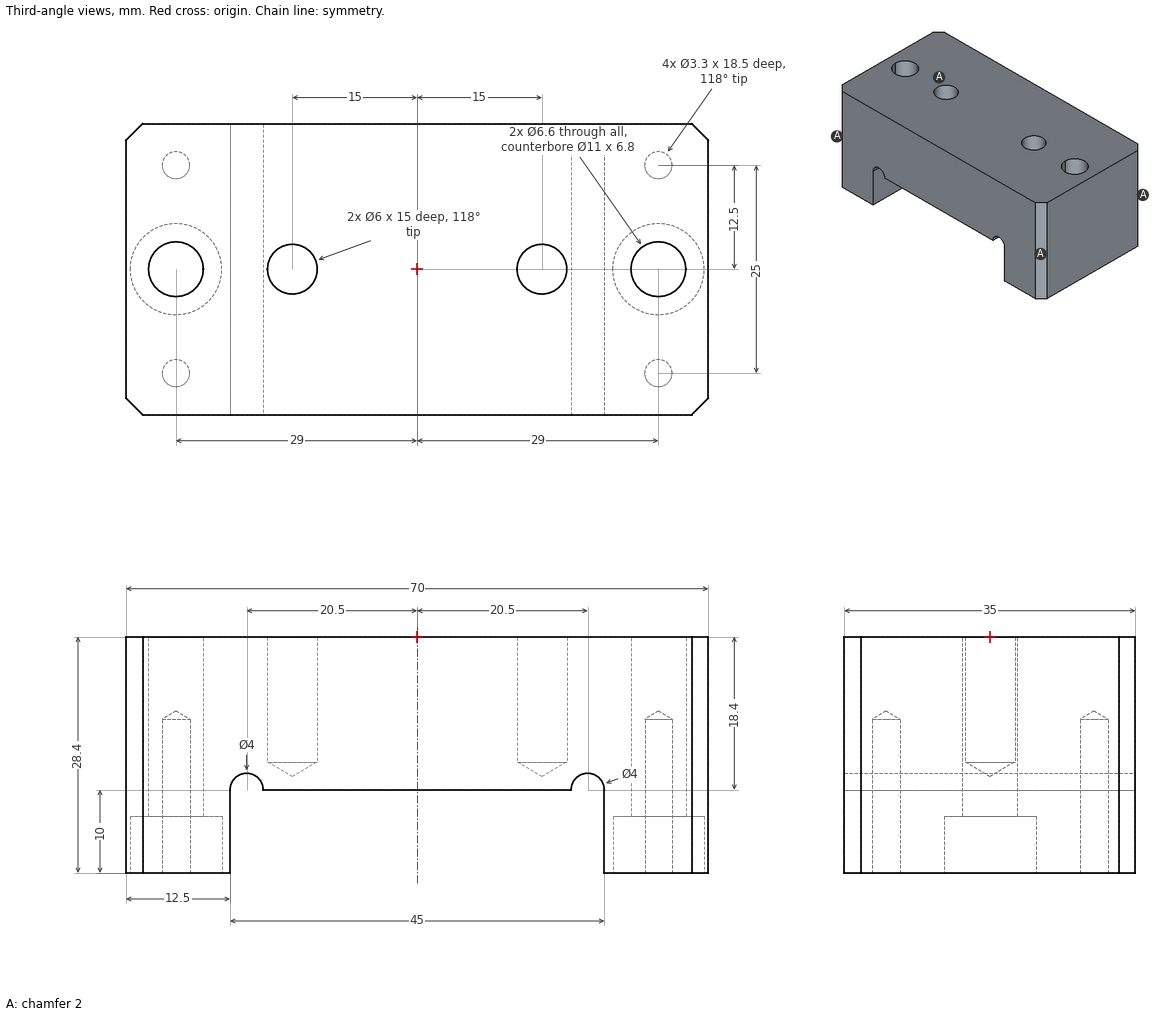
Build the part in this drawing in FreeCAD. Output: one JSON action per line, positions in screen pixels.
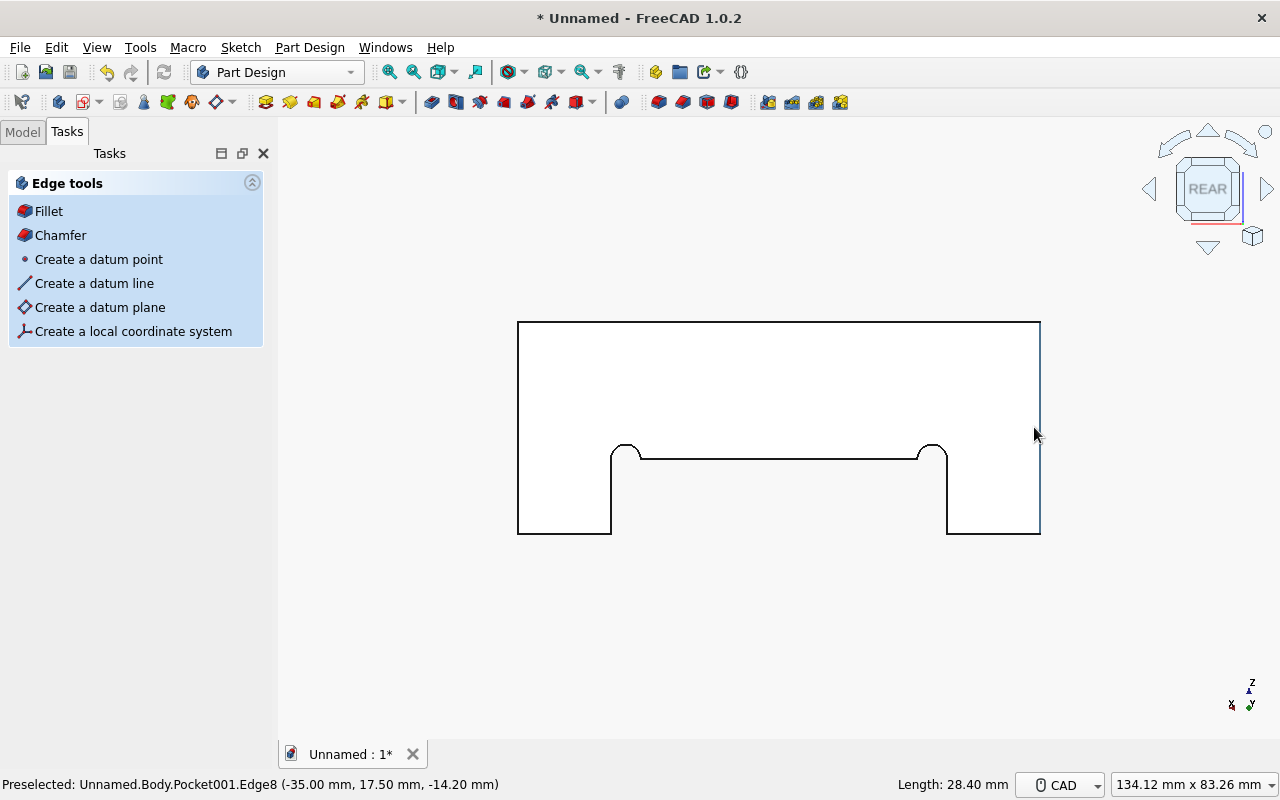
{"action": "key", "text": "0"}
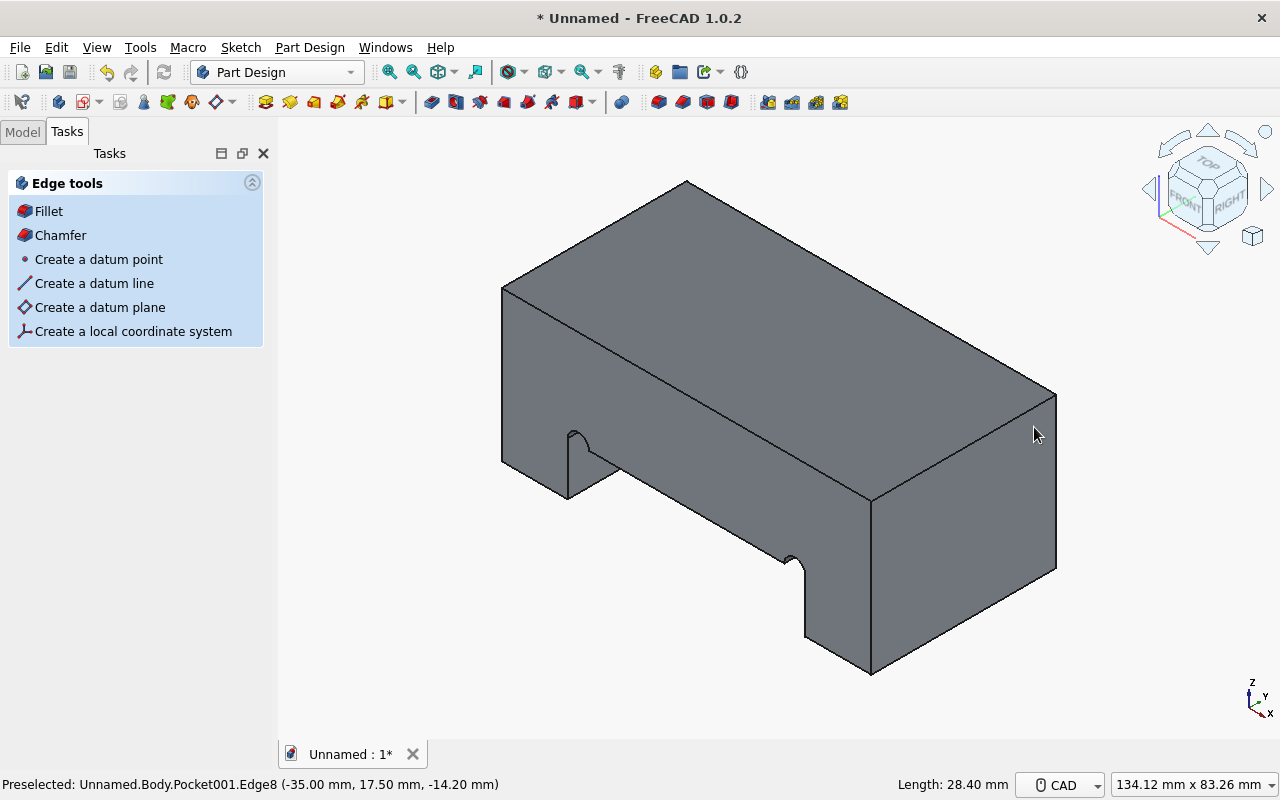
{"action": "left_click", "coordinate": [871, 587], "text": "ctrl"}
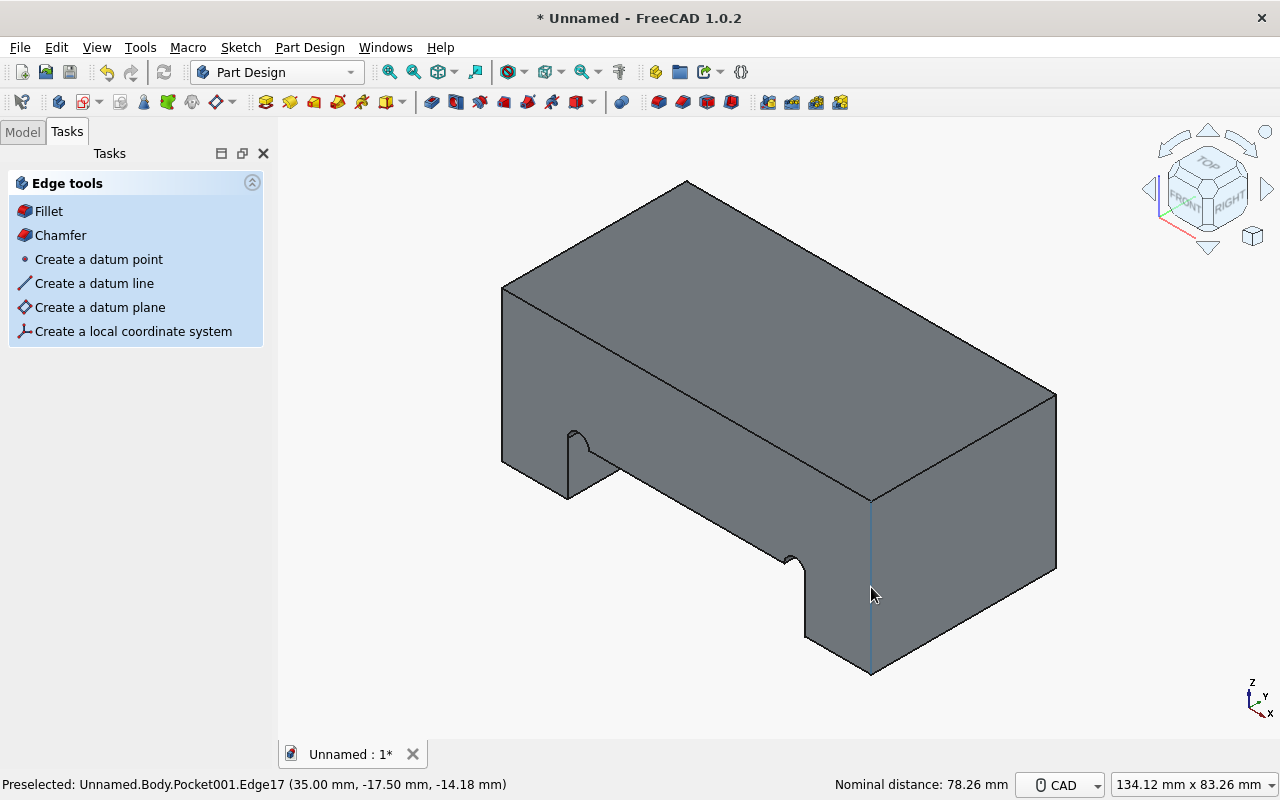
{"action": "key", "text": "2"}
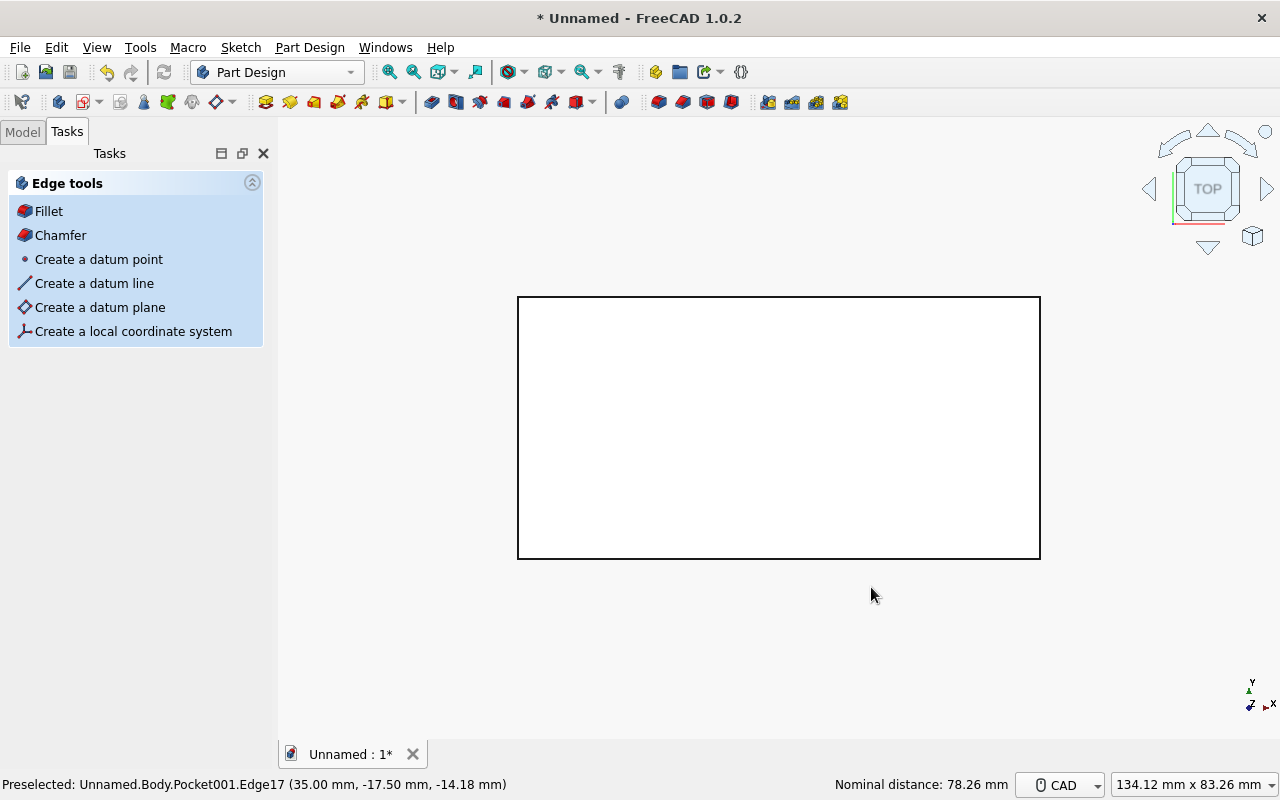
{"action": "key", "text": "1"}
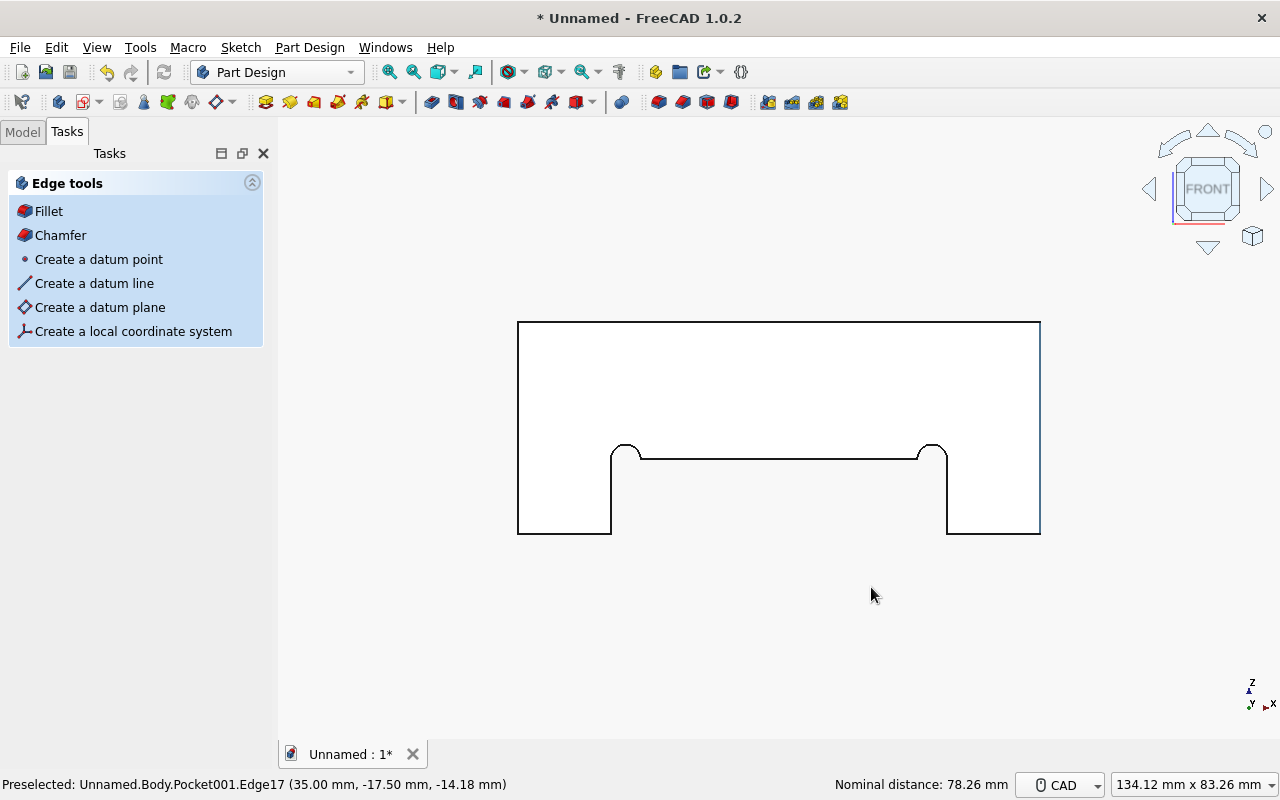
{"action": "left_click", "coordinate": [518, 427], "text": "ctrl"}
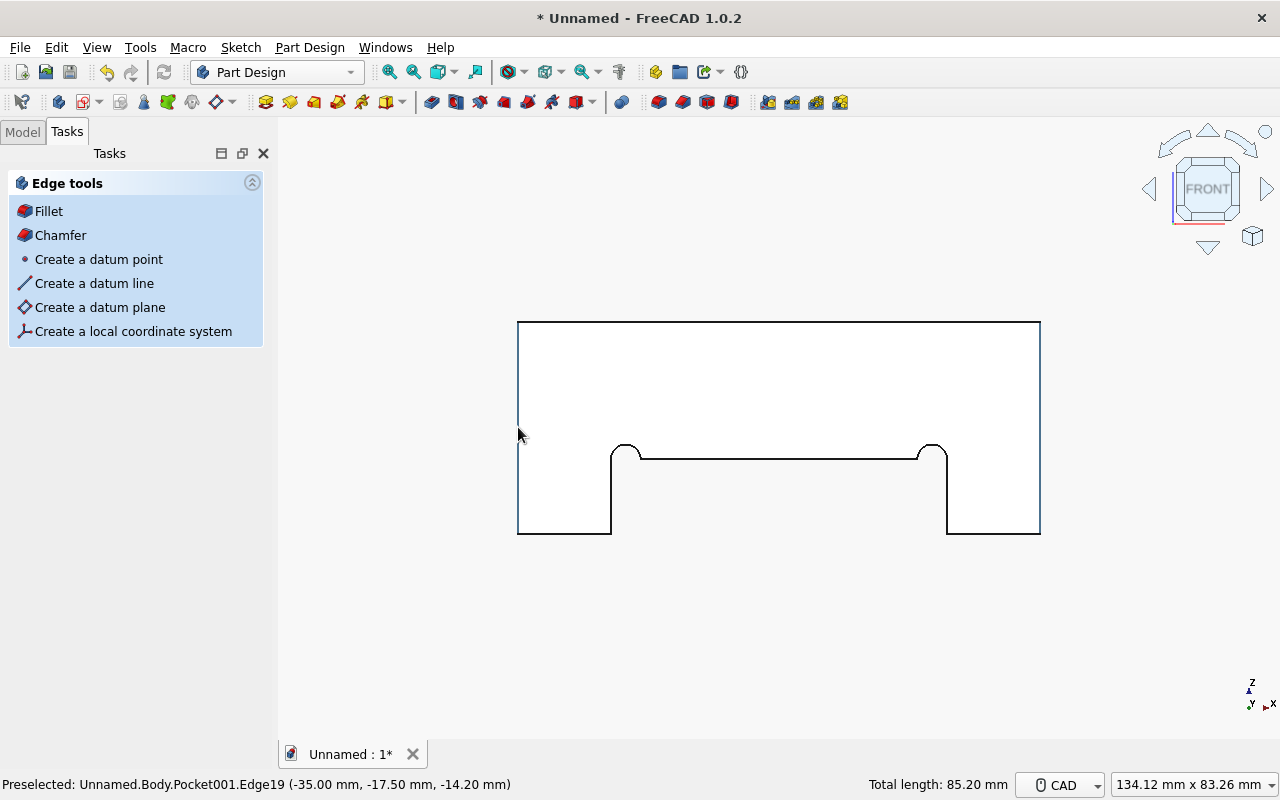
{"action": "key", "text": "3"}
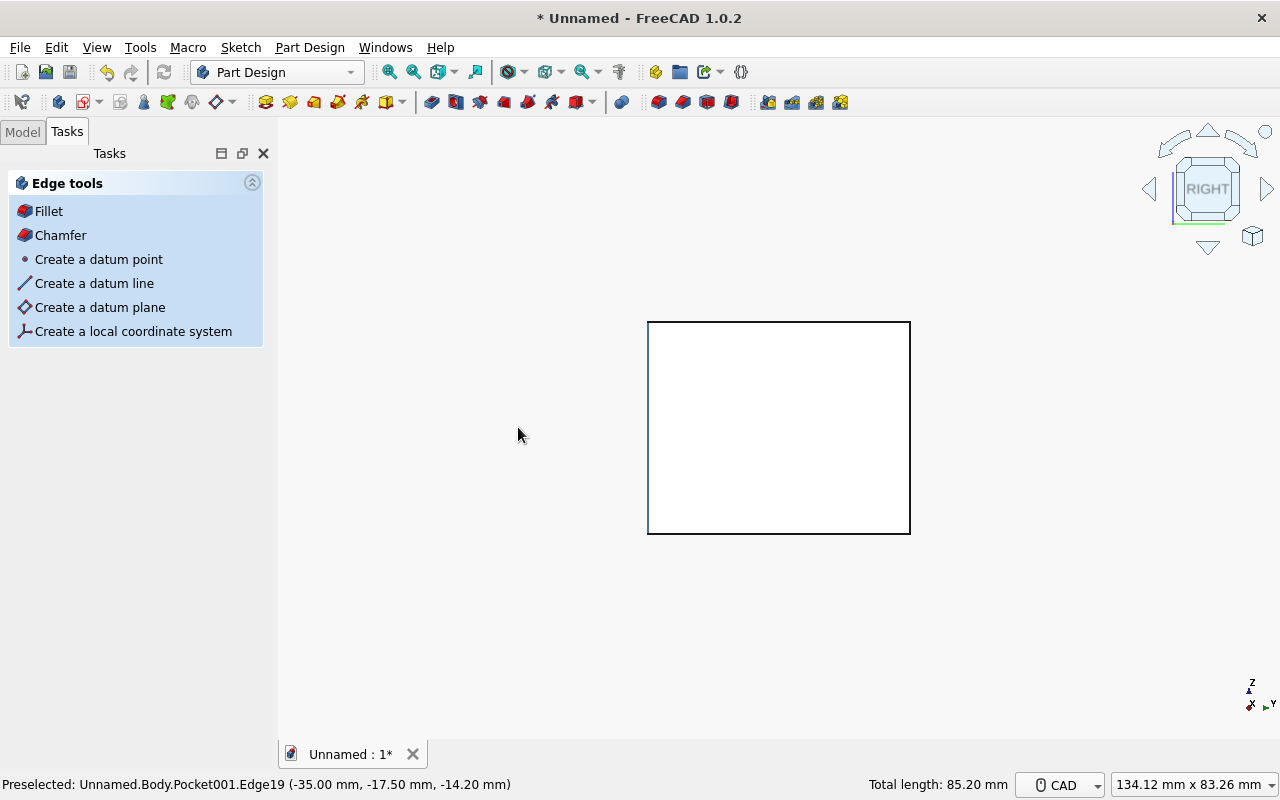
{"action": "key", "text": "v f"}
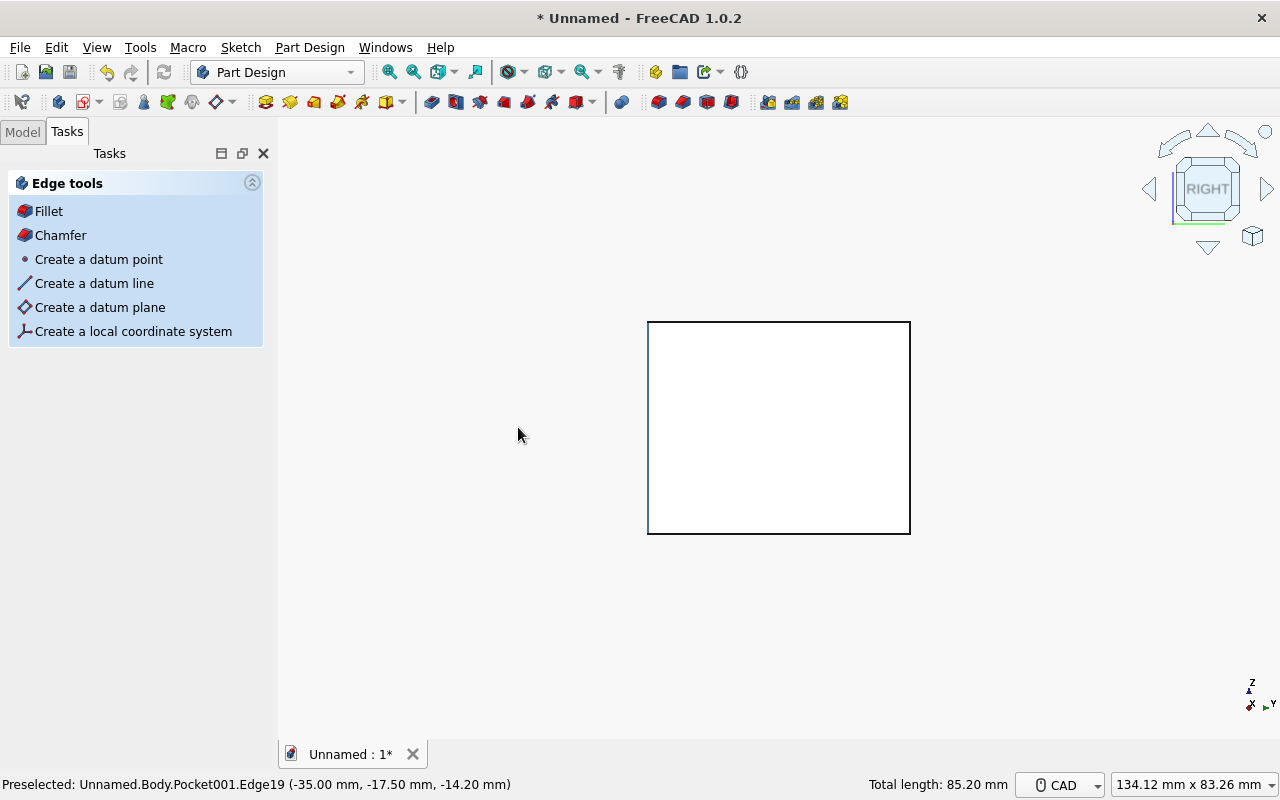
{"action": "left_click", "coordinate": [910, 427], "text": "ctrl"}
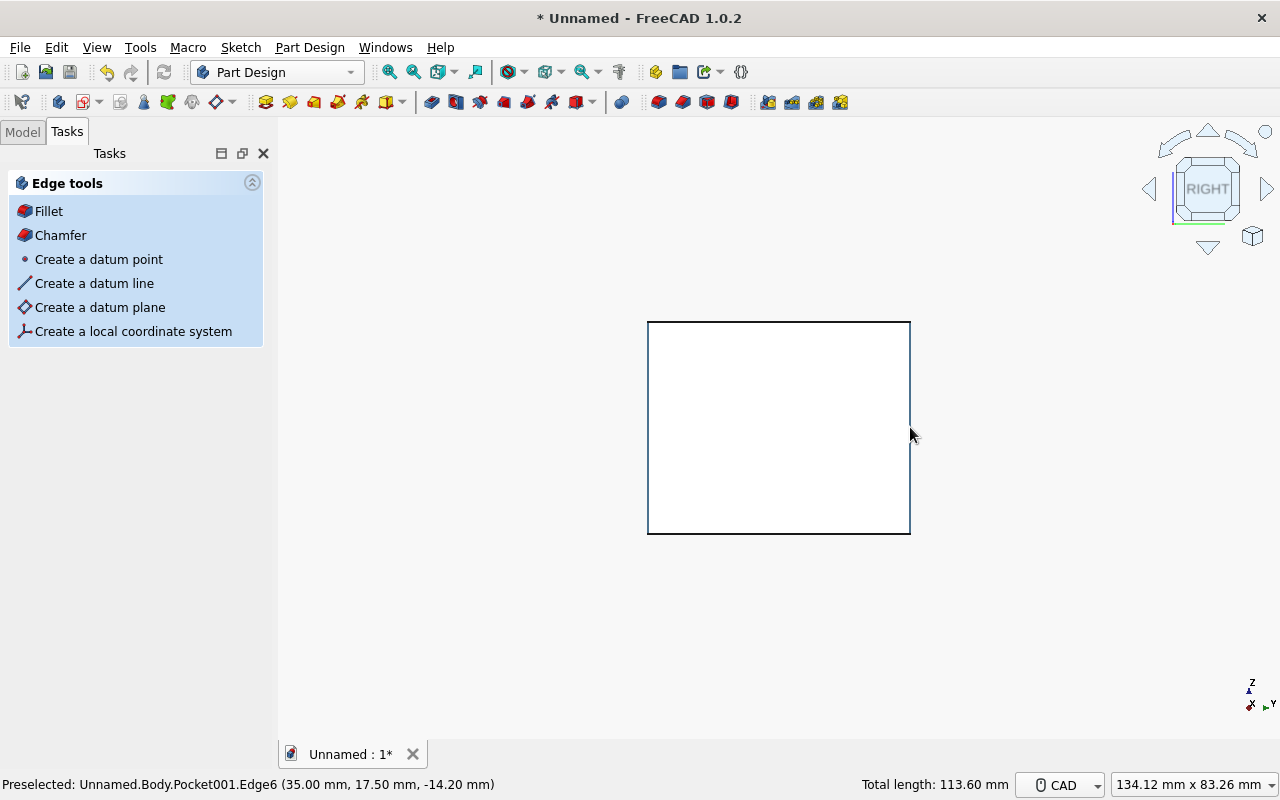
{"action": "left_click", "coordinate": [684, 102]}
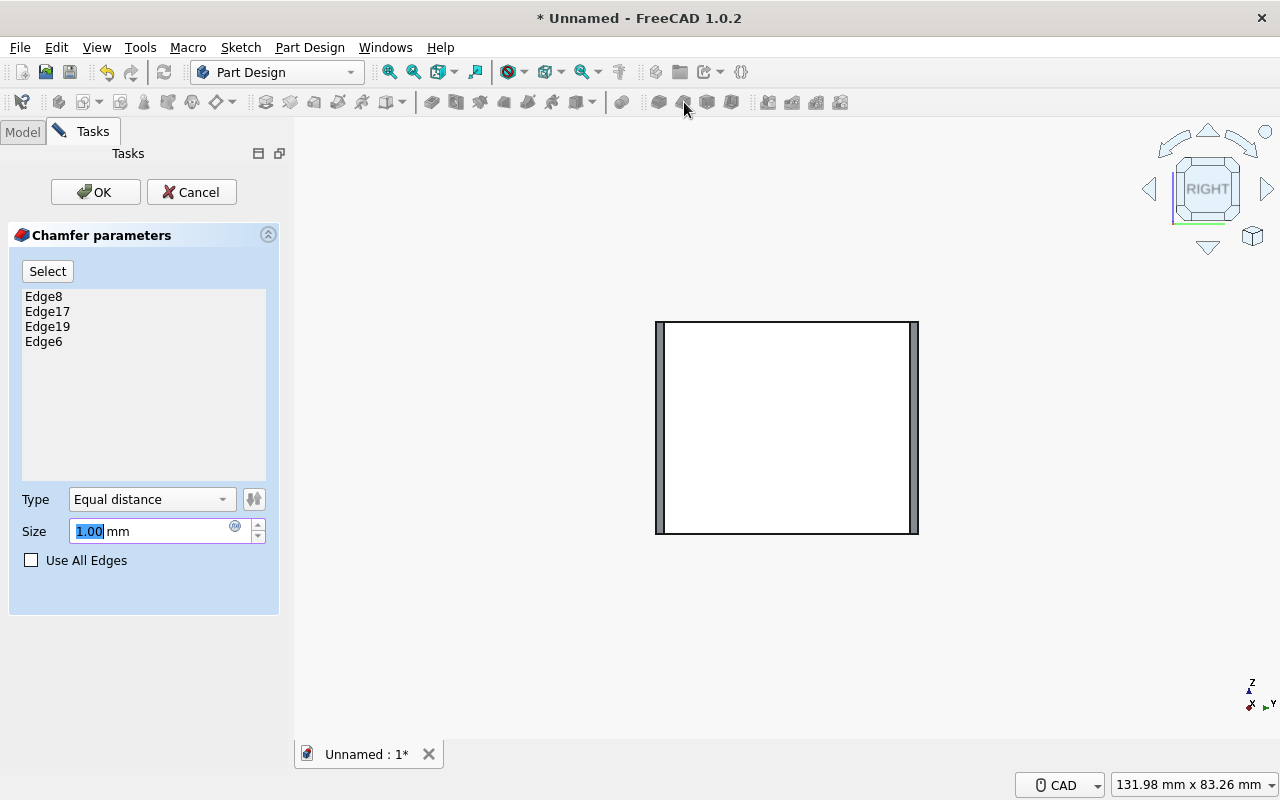
{"action": "type", "text": "2"}
{"action": "key", "text": "Tab"}